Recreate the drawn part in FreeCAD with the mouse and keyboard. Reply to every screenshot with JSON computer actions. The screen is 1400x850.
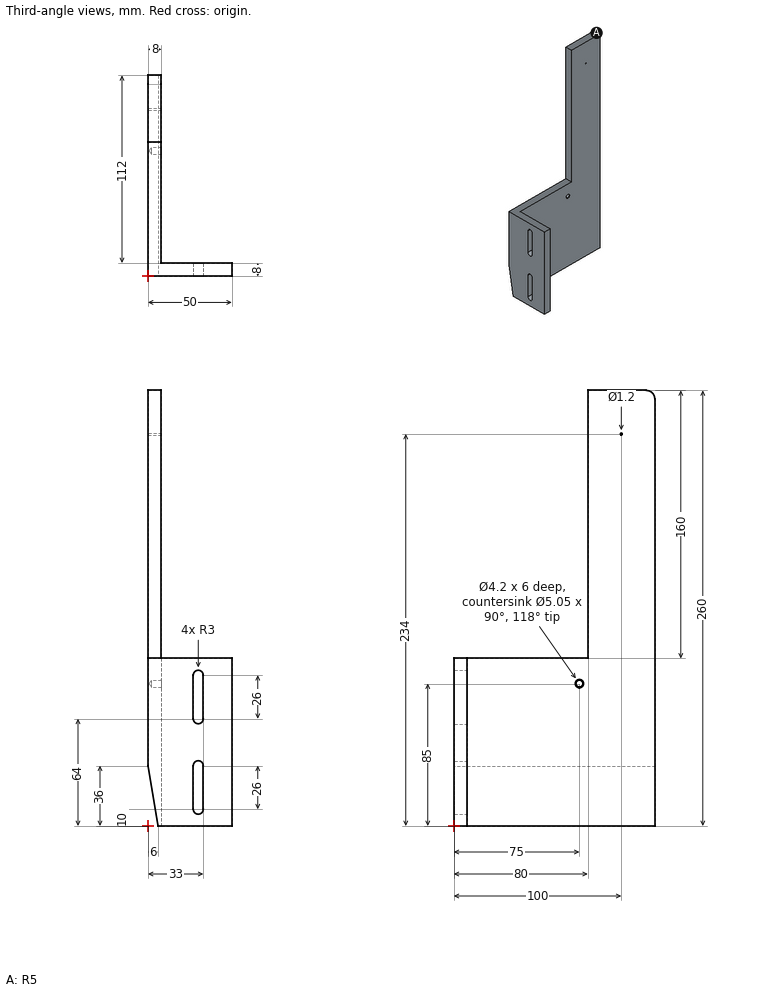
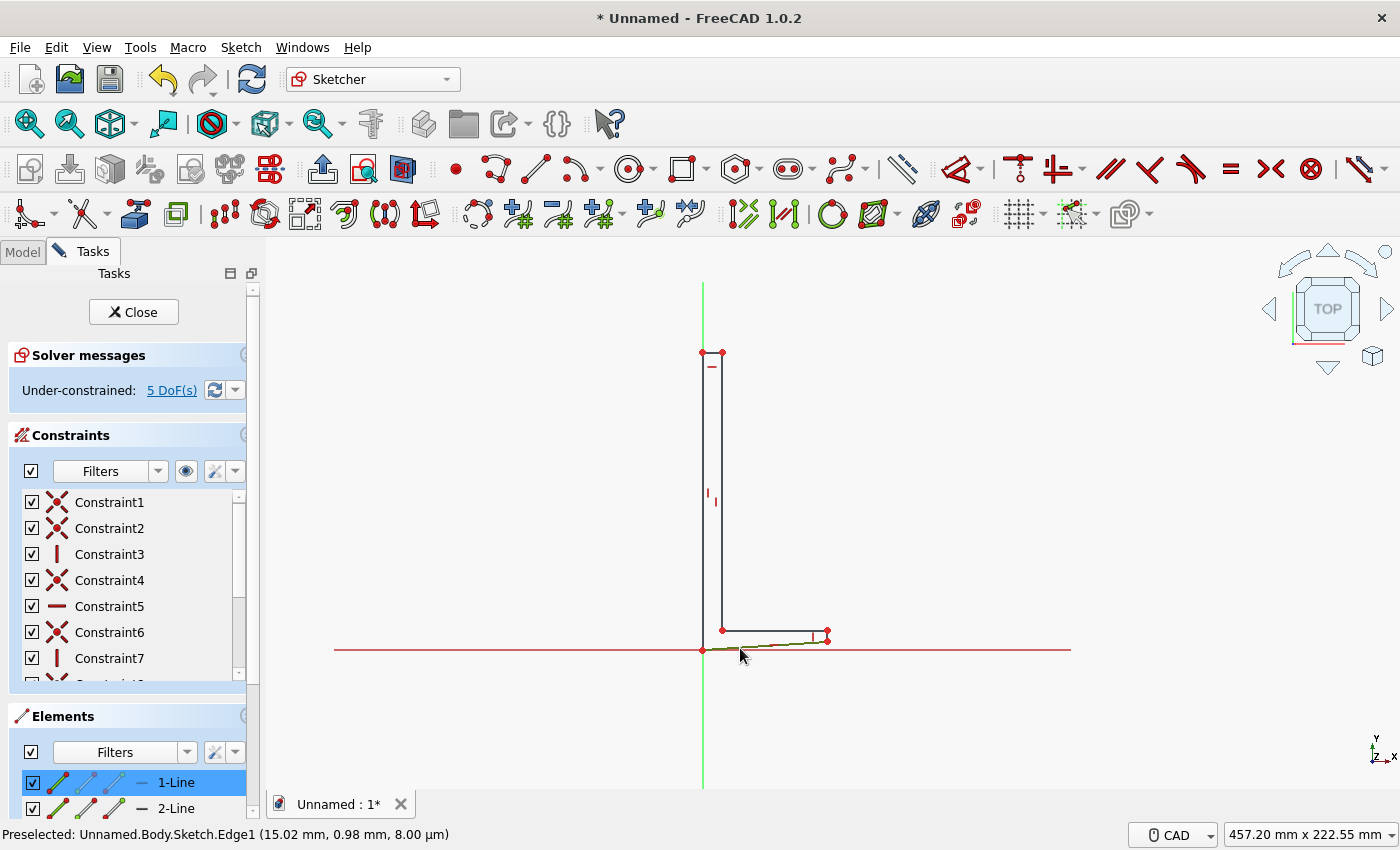
{"action": "key", "text": "h"}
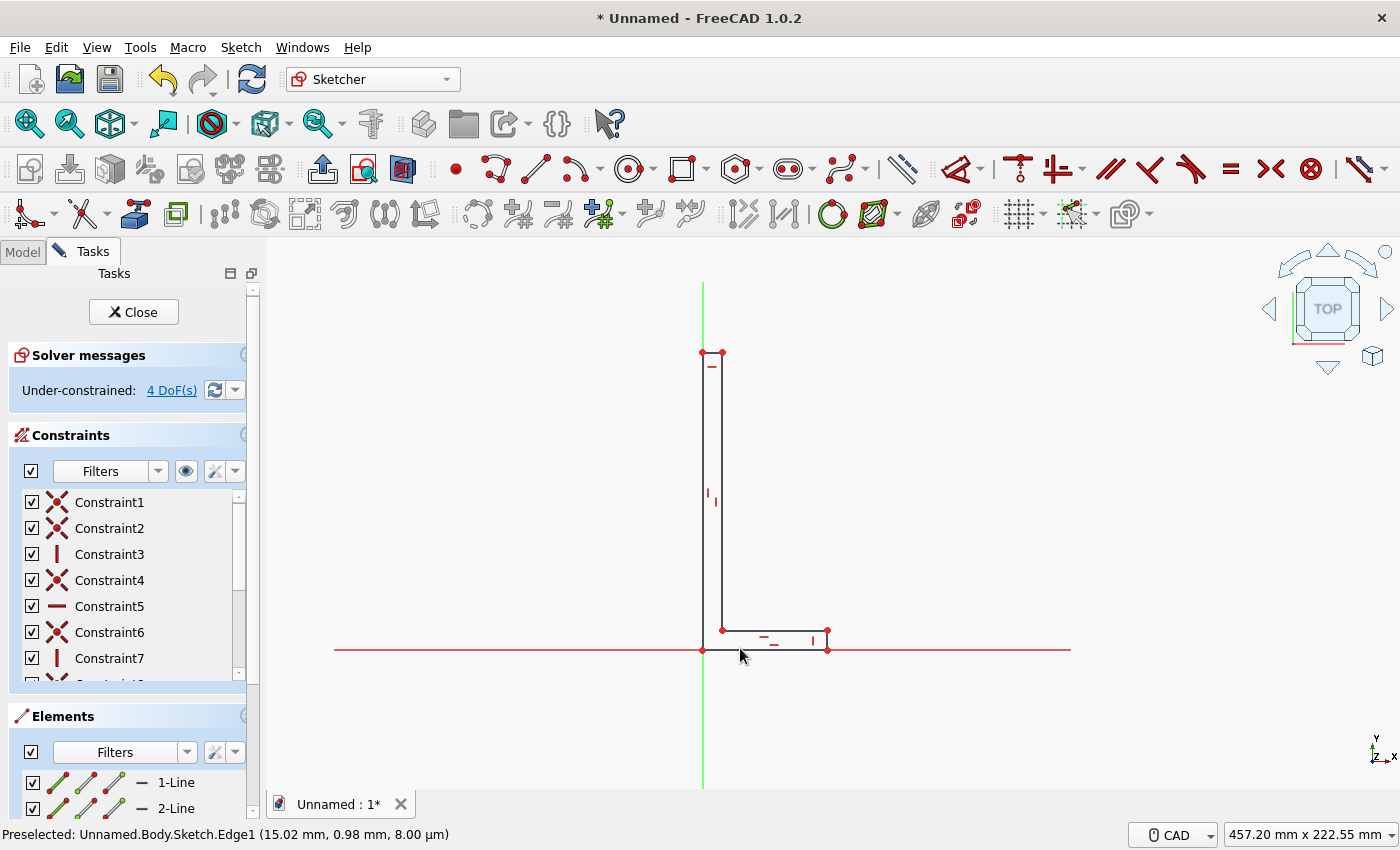
{"action": "left_click", "coordinate": [956, 170]}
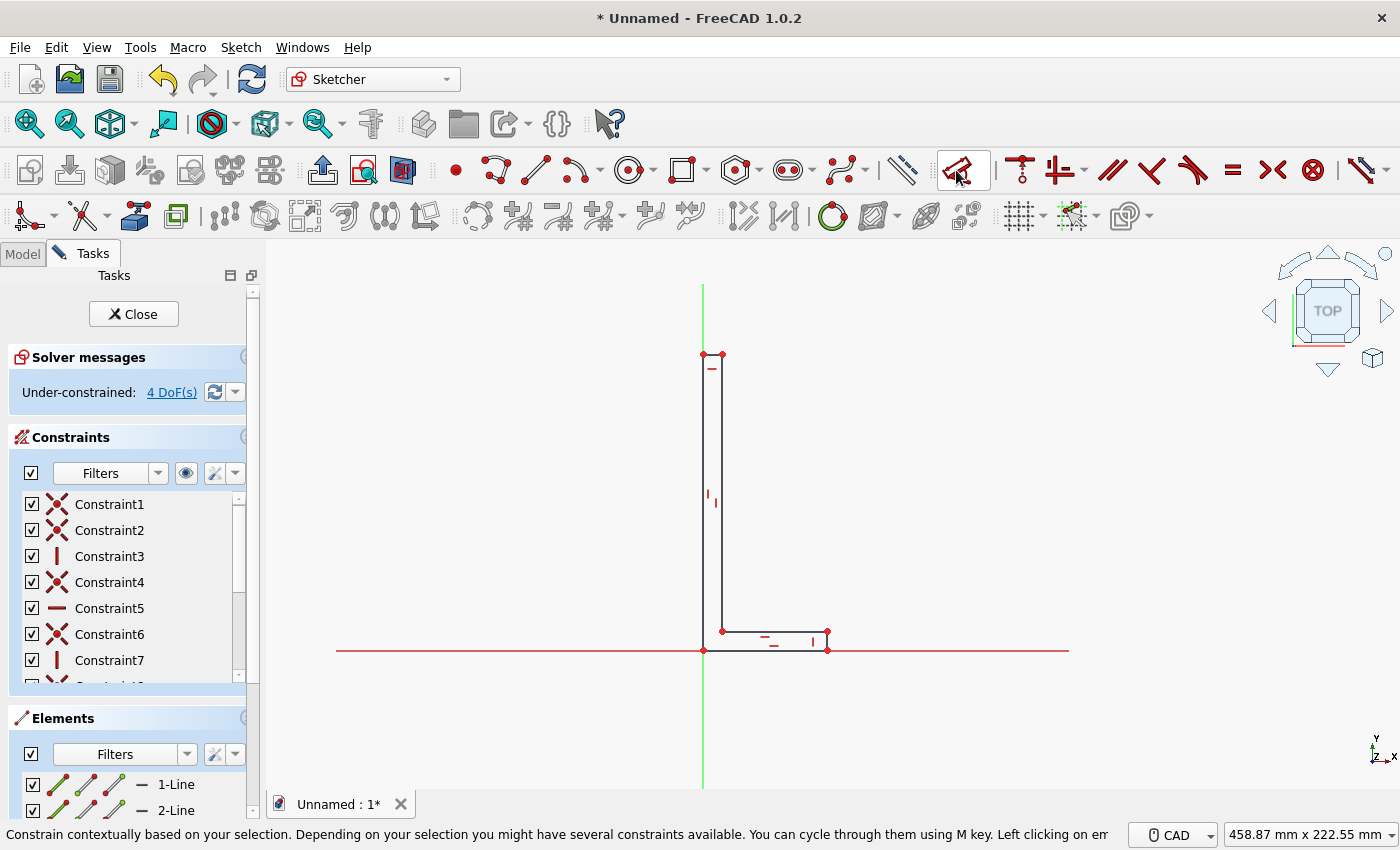
{"action": "scroll", "coordinate": [827, 641], "scroll_direction": "up", "scroll_amount": 4}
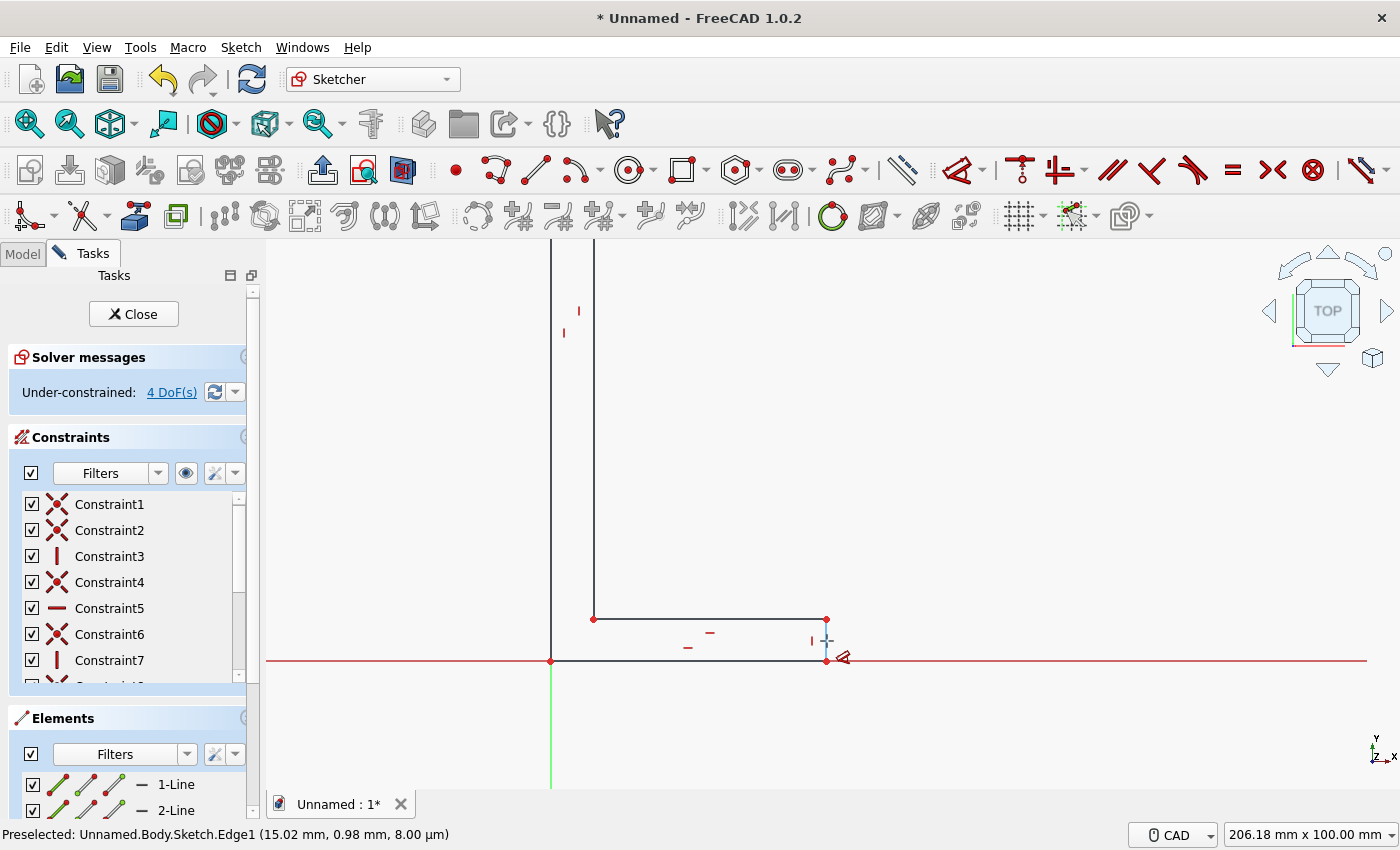
{"action": "left_click", "coordinate": [826, 640]}
{"action": "left_click", "coordinate": [860, 640]}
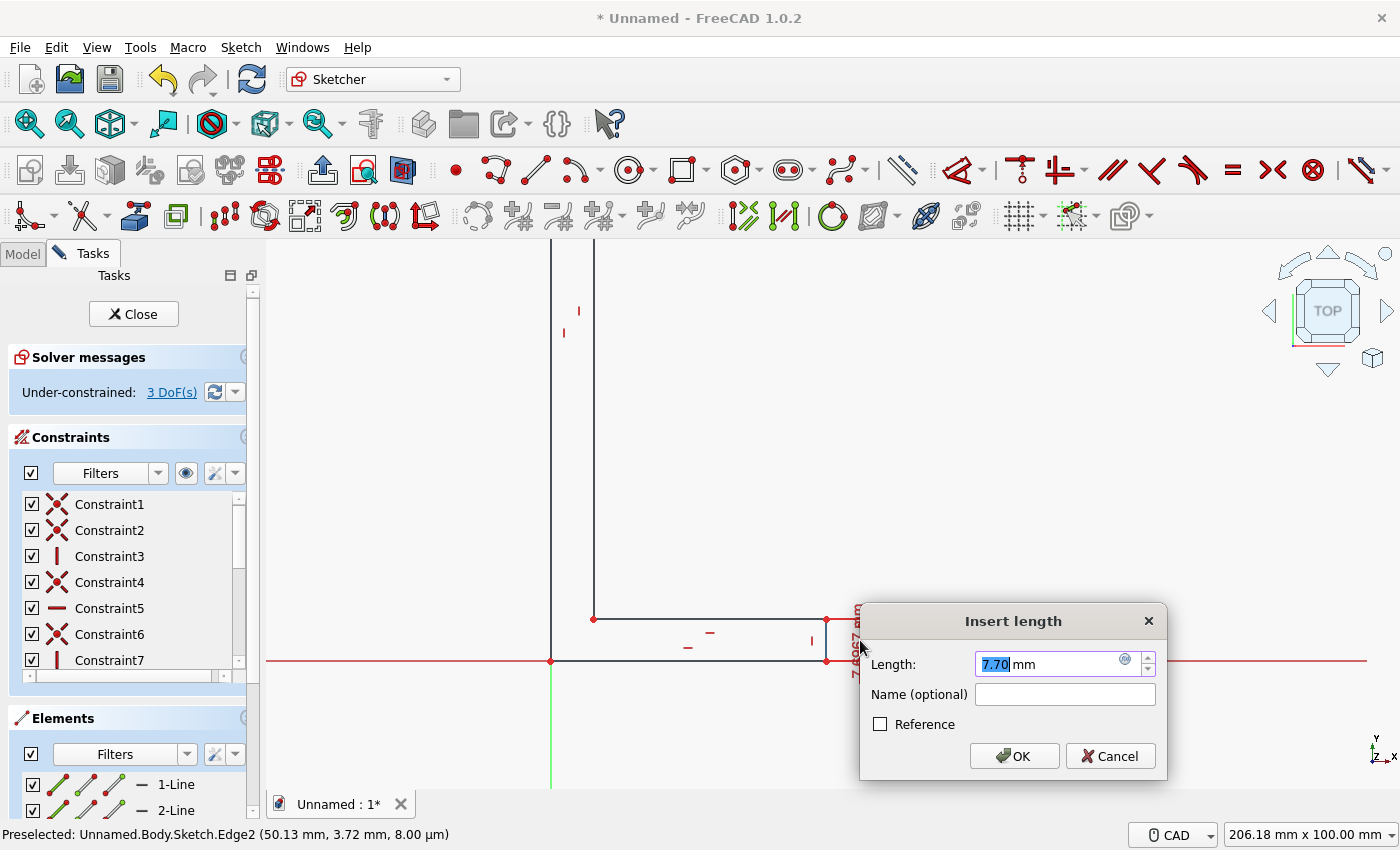
{"action": "type", "text": "8"}
{"action": "key", "text": "Return"}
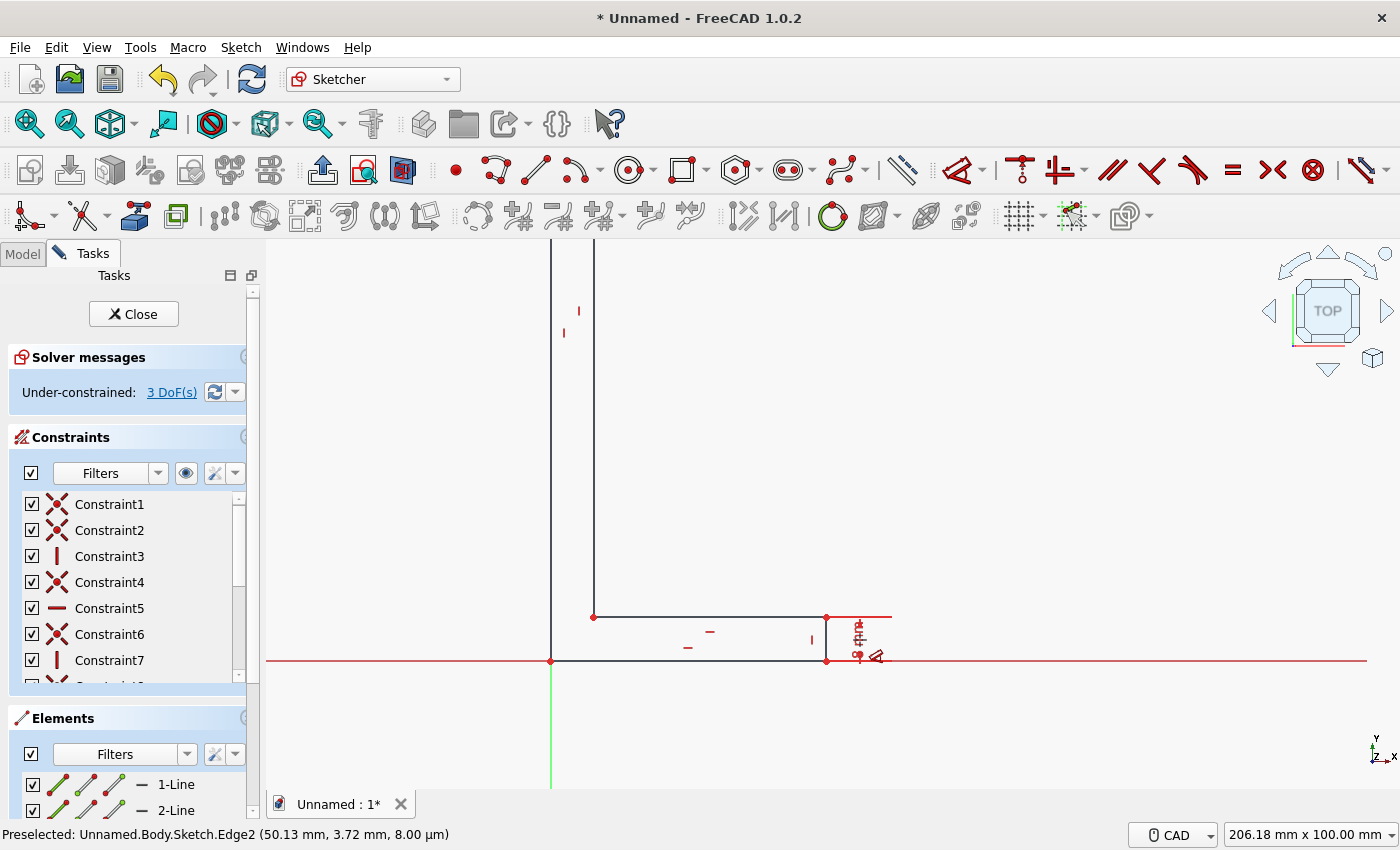
{"action": "scroll", "coordinate": [857, 736], "scroll_direction": "down", "scroll_amount": 3}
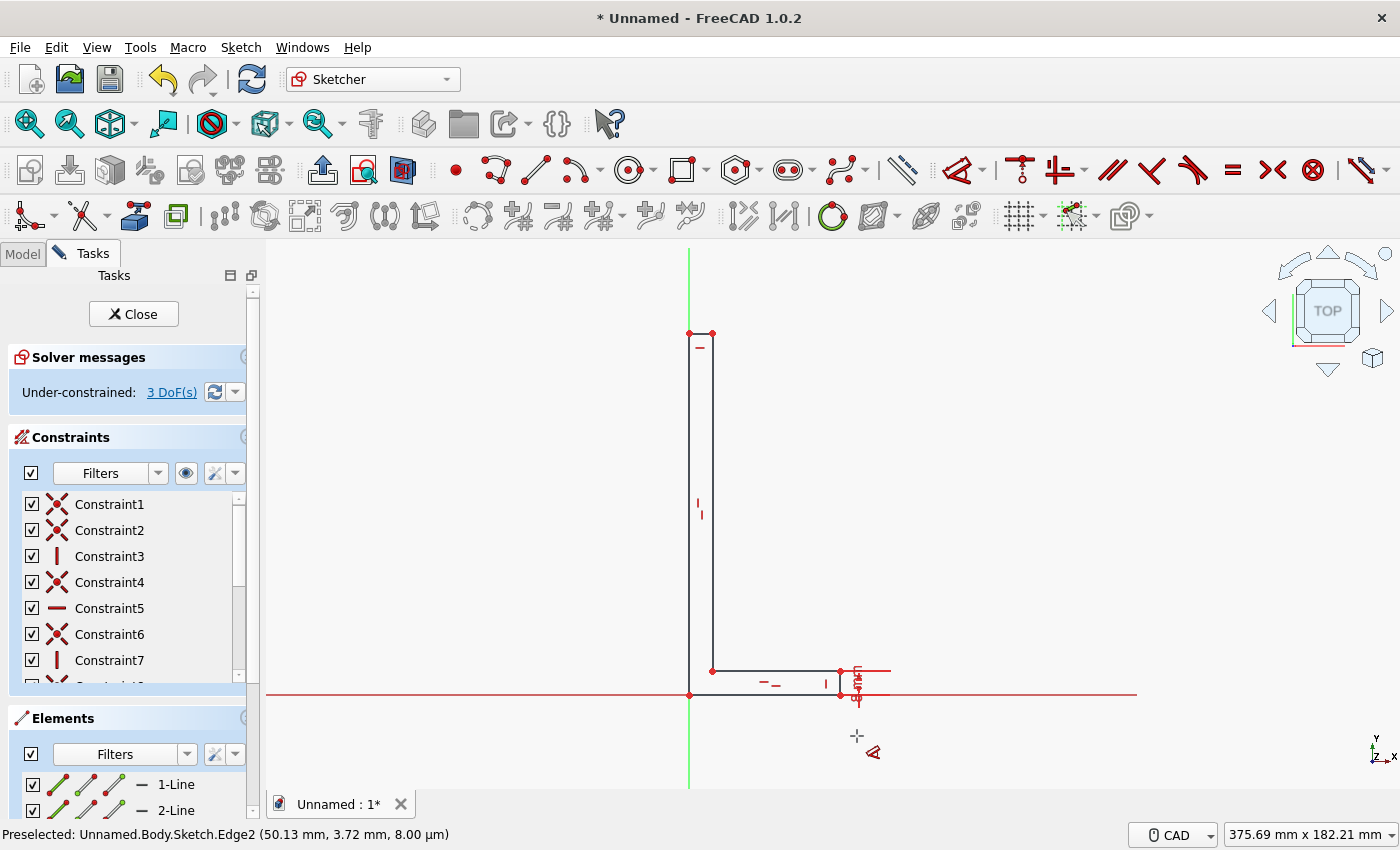
{"action": "scroll", "coordinate": [706, 334], "scroll_direction": "up", "scroll_amount": 4}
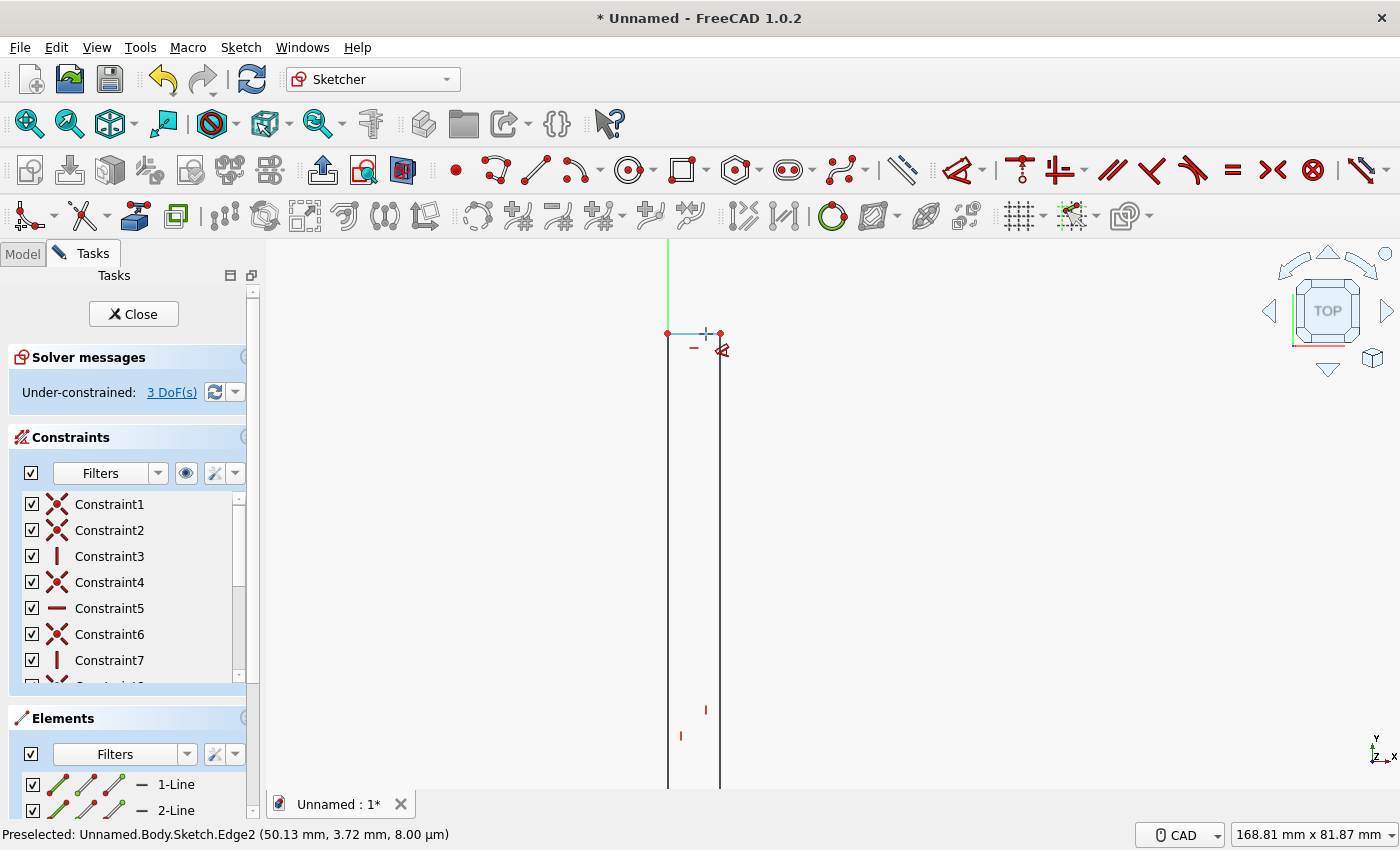
{"action": "left_click", "coordinate": [705, 334]}
{"action": "left_click", "coordinate": [694, 300]}